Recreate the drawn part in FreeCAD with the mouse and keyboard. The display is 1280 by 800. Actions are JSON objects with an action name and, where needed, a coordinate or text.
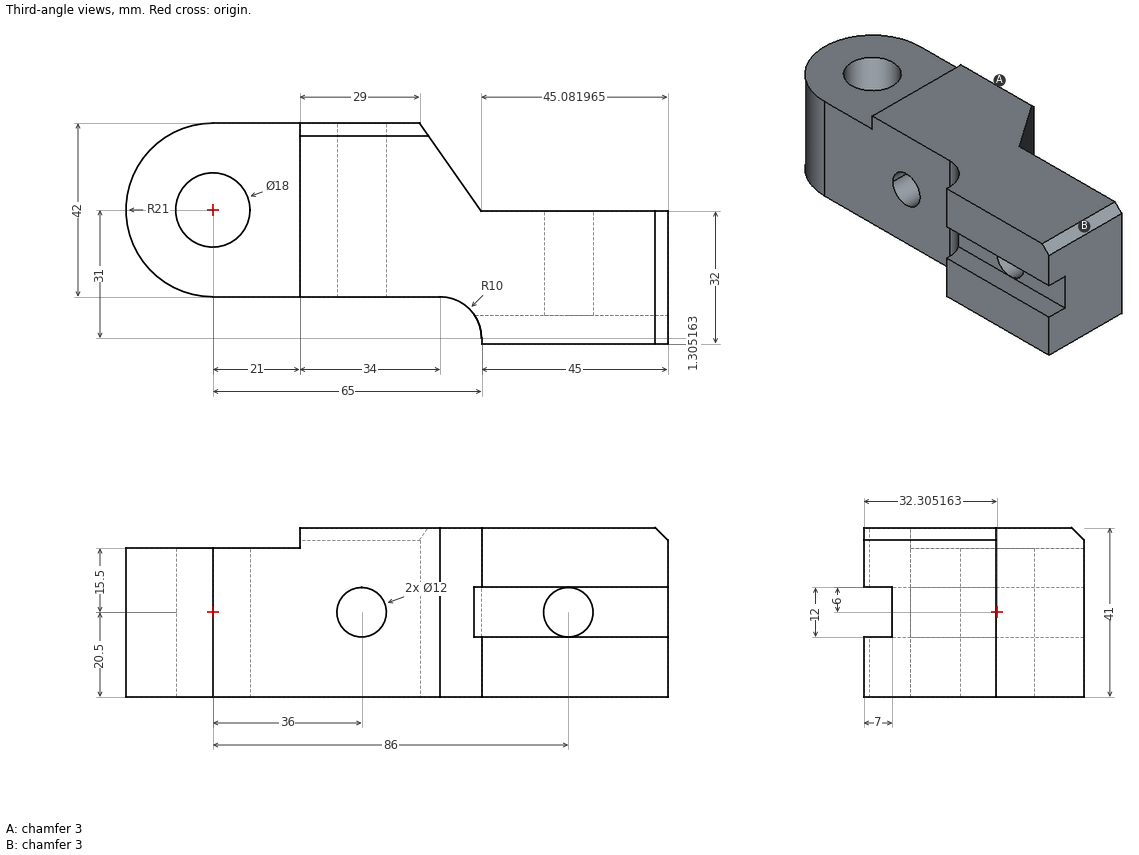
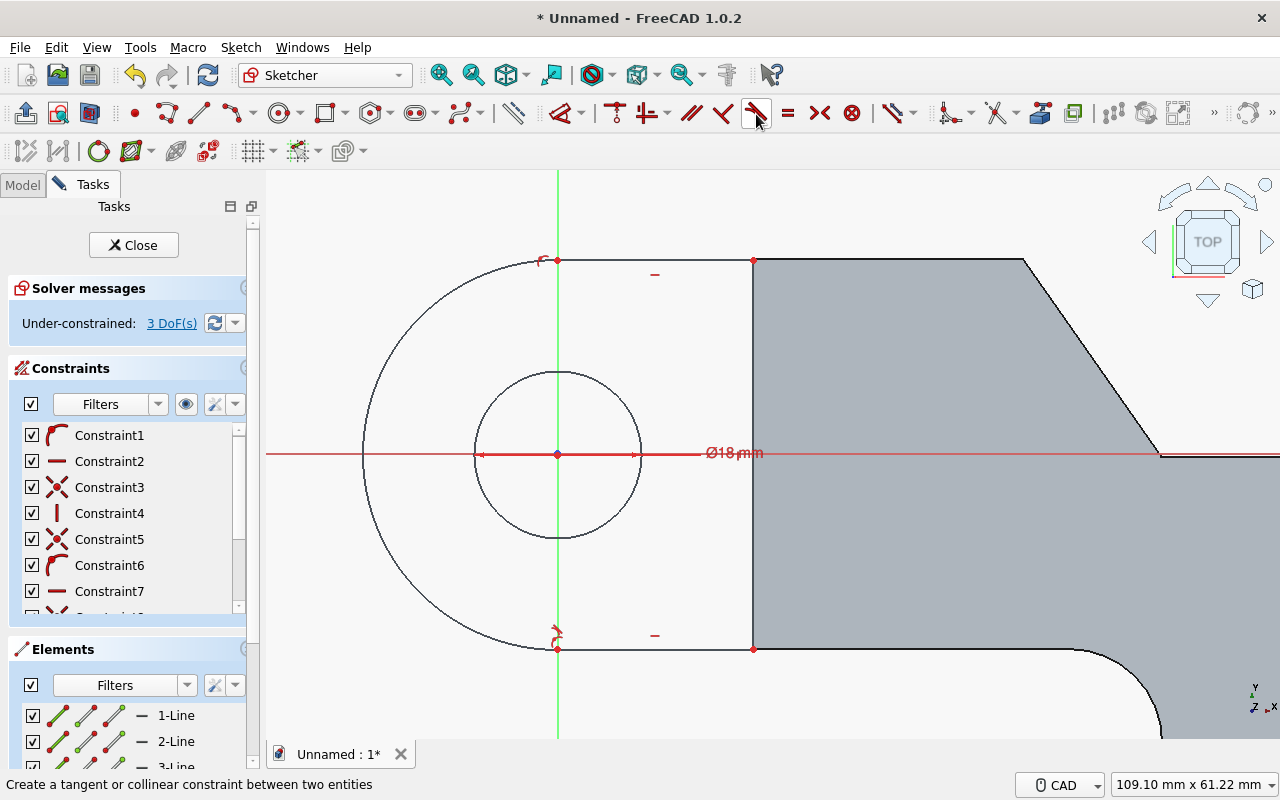
{"action": "left_click", "coordinate": [558, 455]}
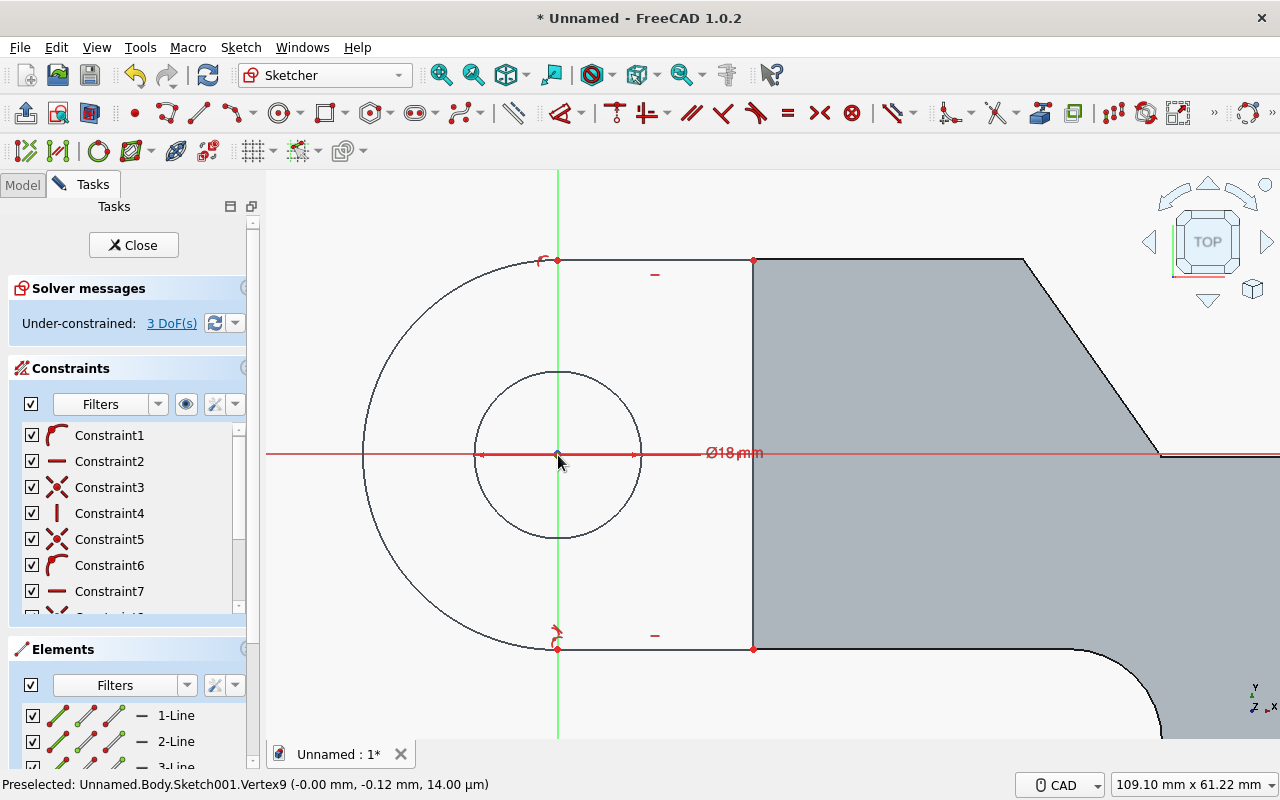
{"action": "left_click", "coordinate": [411, 454]}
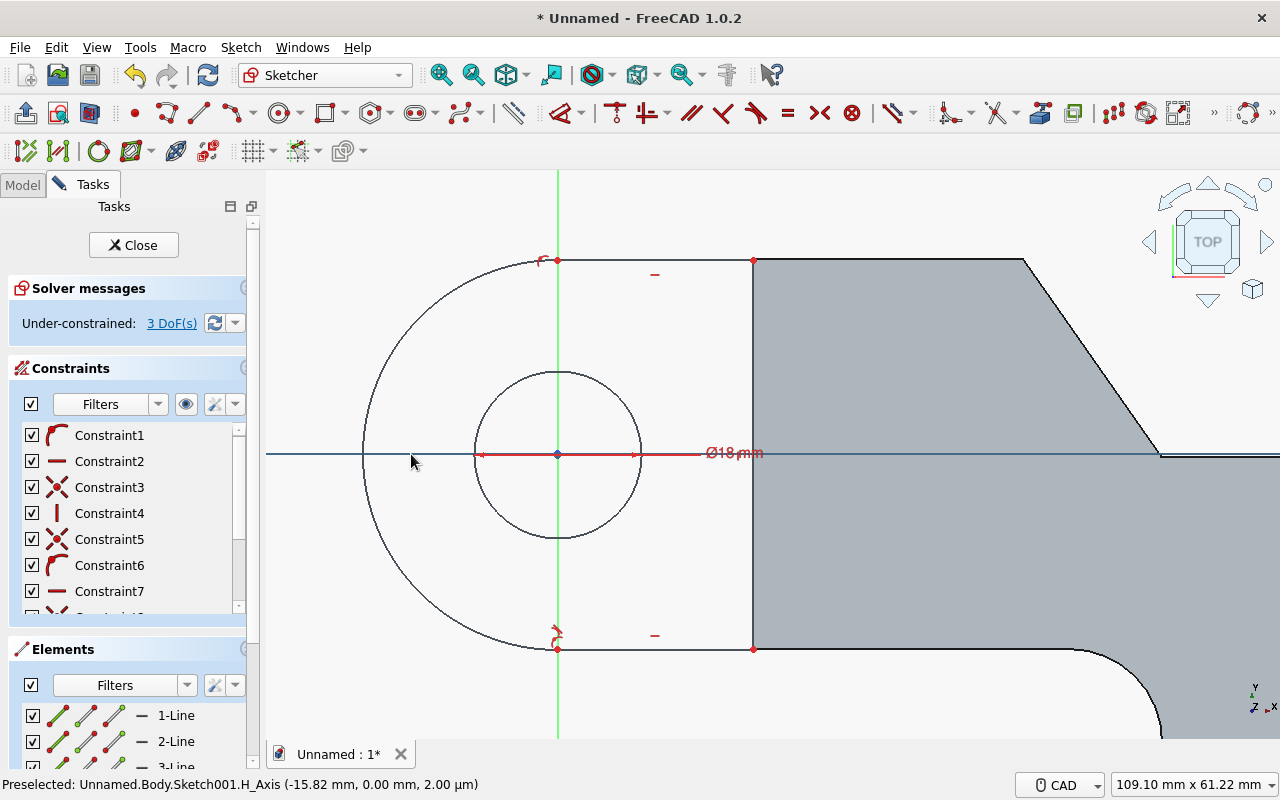
{"action": "left_click", "coordinate": [616, 114]}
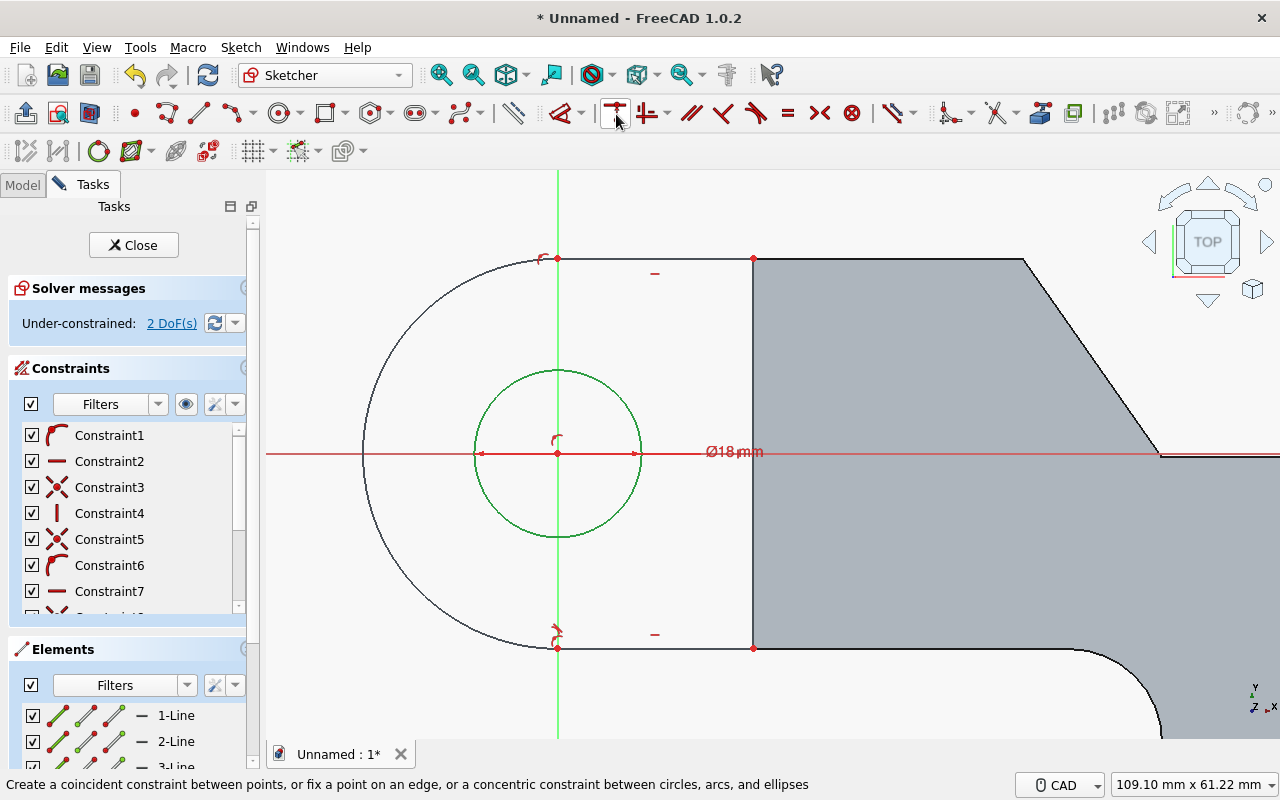
{"action": "left_click", "coordinate": [560, 114]}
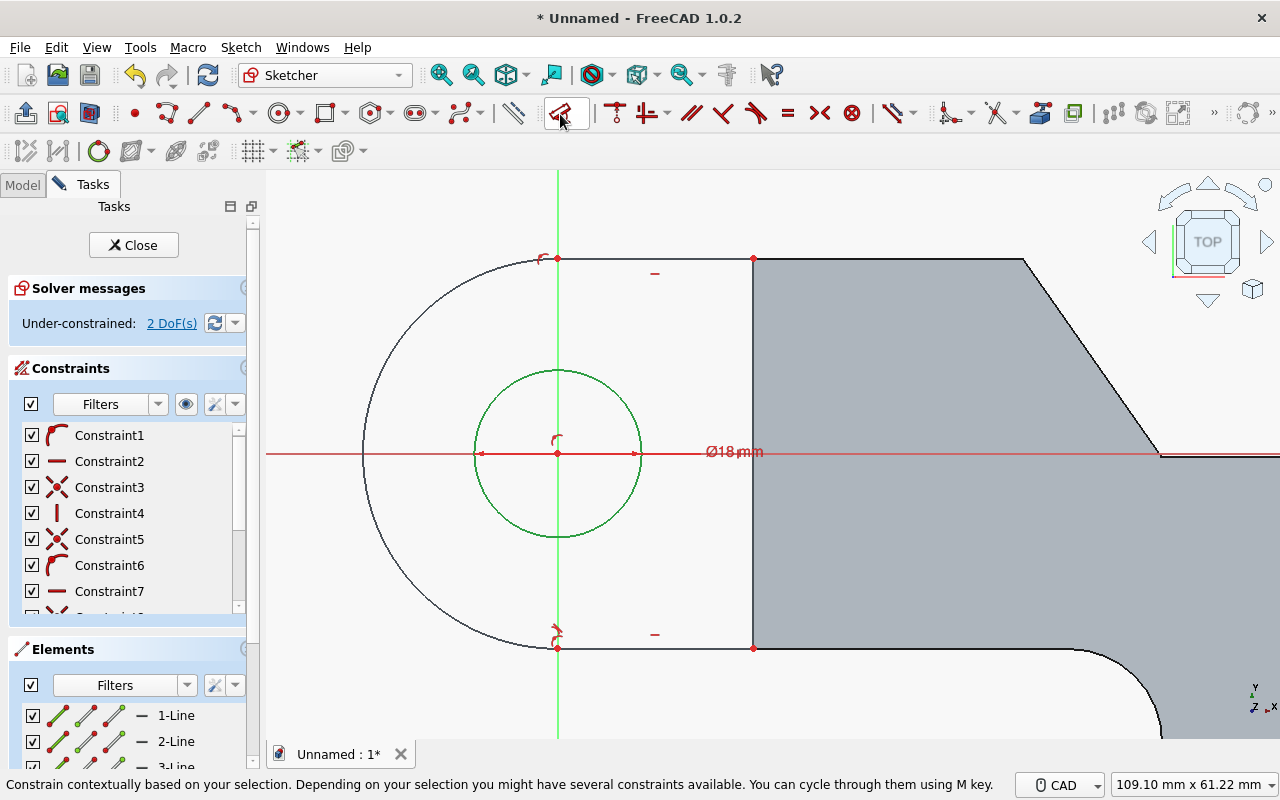
{"action": "left_click", "coordinate": [400, 339]}
{"action": "left_click", "coordinate": [374, 320]}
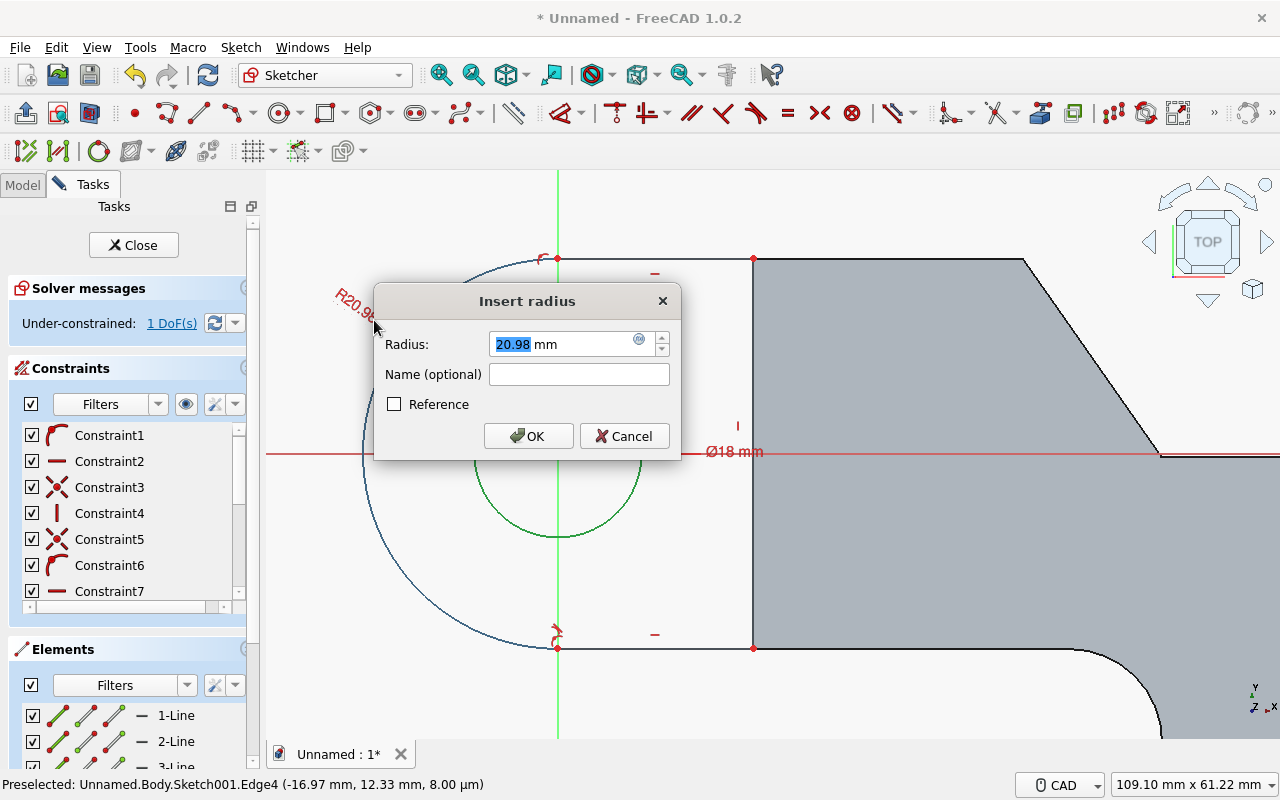
{"action": "type", "text": "21"}
{"action": "key", "text": "Return"}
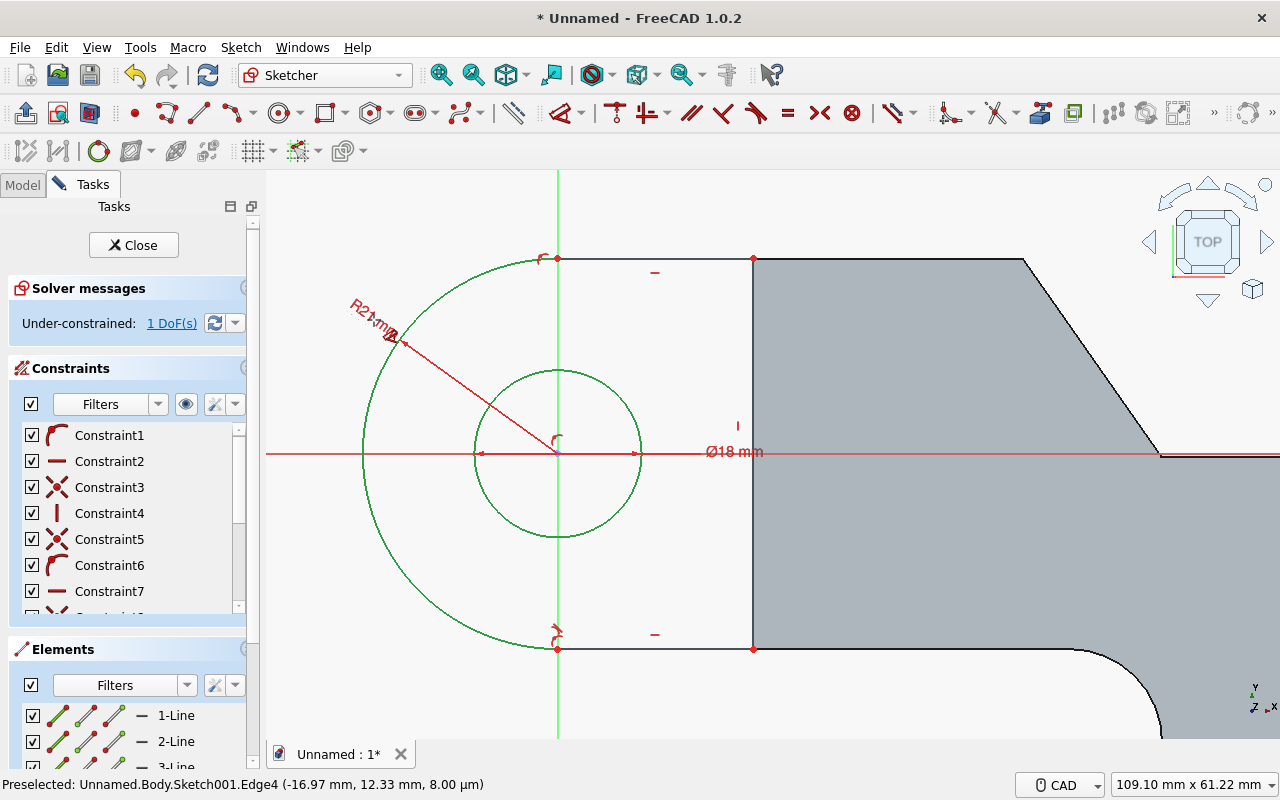
{"action": "left_click", "coordinate": [616, 649]}
{"action": "left_click", "coordinate": [655, 683]}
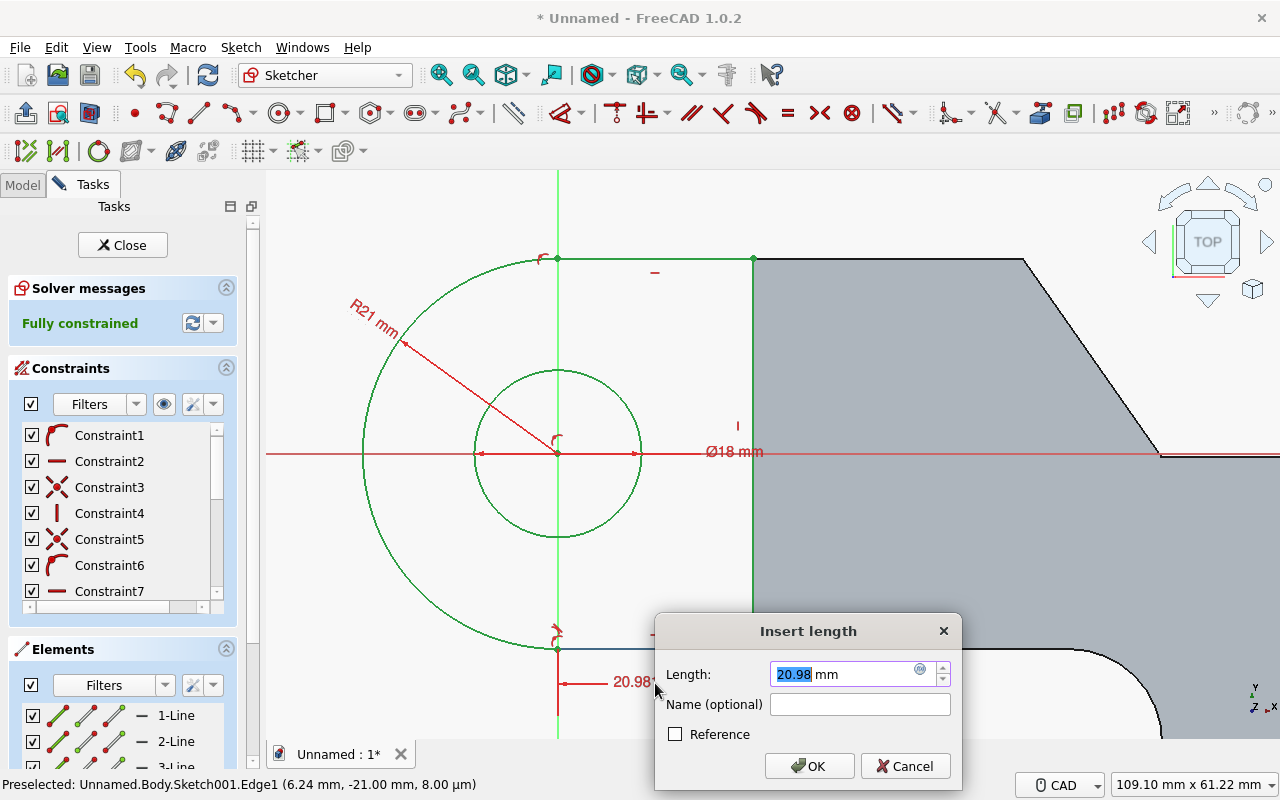
{"action": "type", "text": "21"}
{"action": "key", "text": "Return"}
{"action": "key", "text": "Escape"}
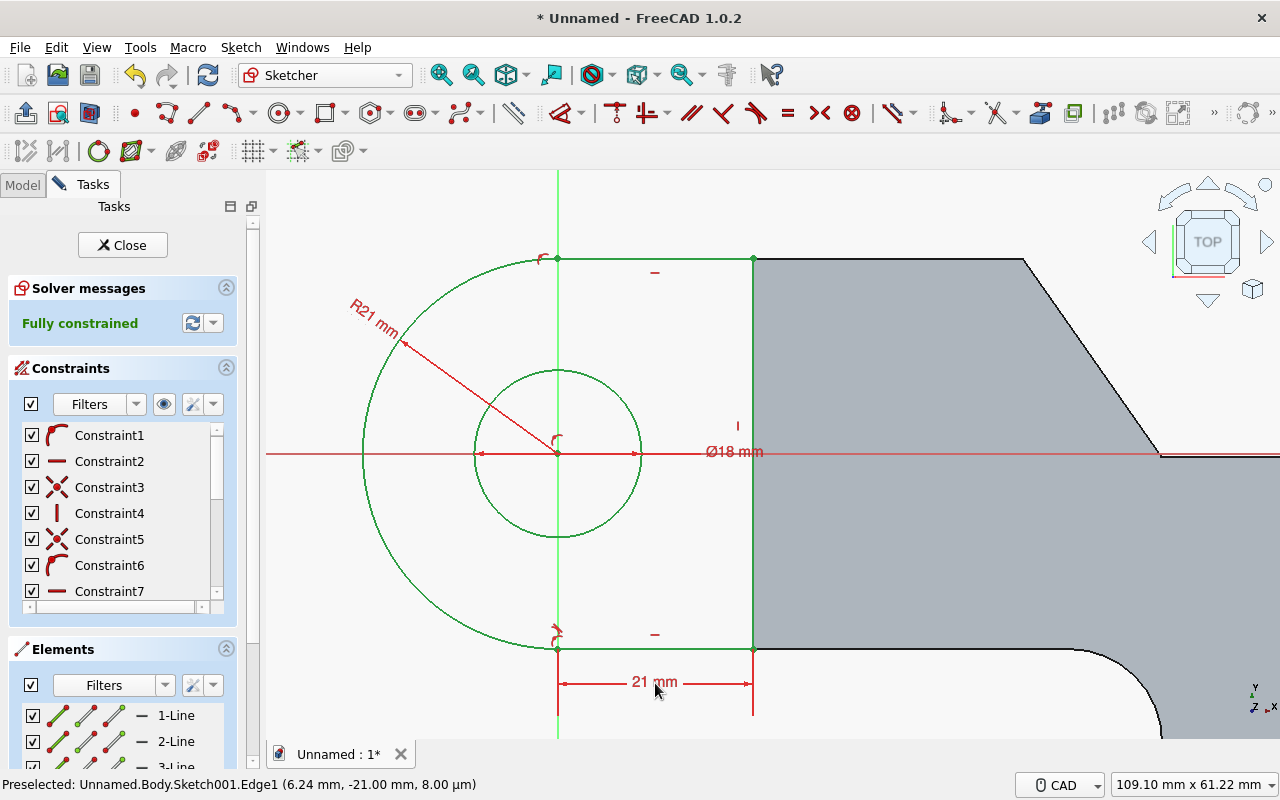
{"action": "left_click", "coordinate": [123, 245]}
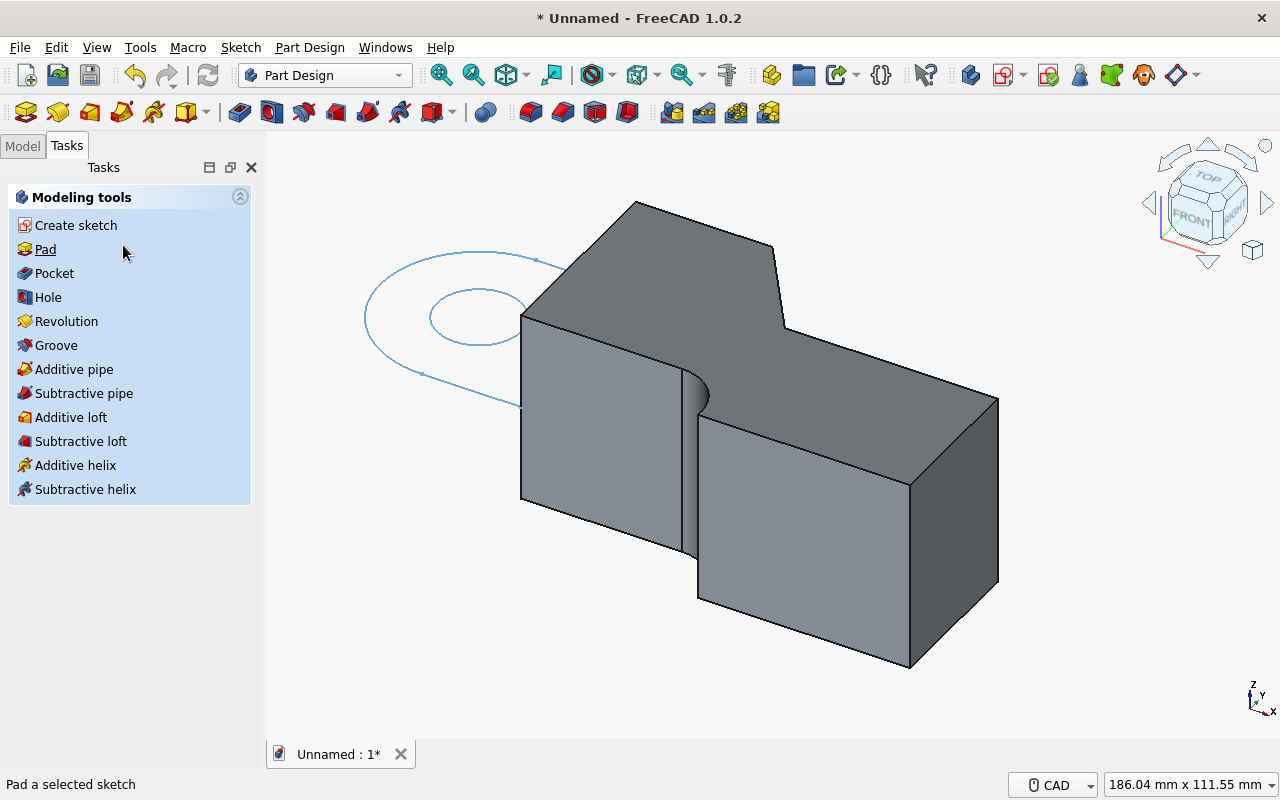
{"action": "left_click", "coordinate": [26, 112]}